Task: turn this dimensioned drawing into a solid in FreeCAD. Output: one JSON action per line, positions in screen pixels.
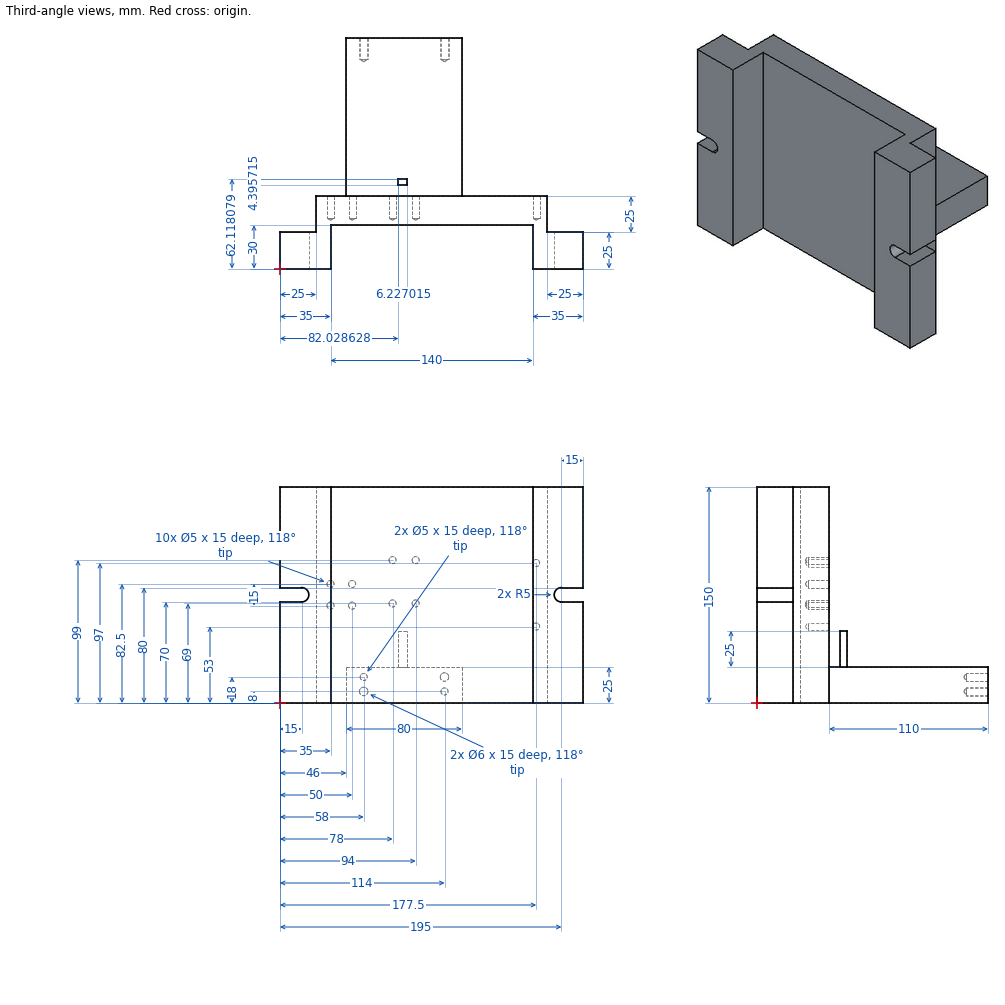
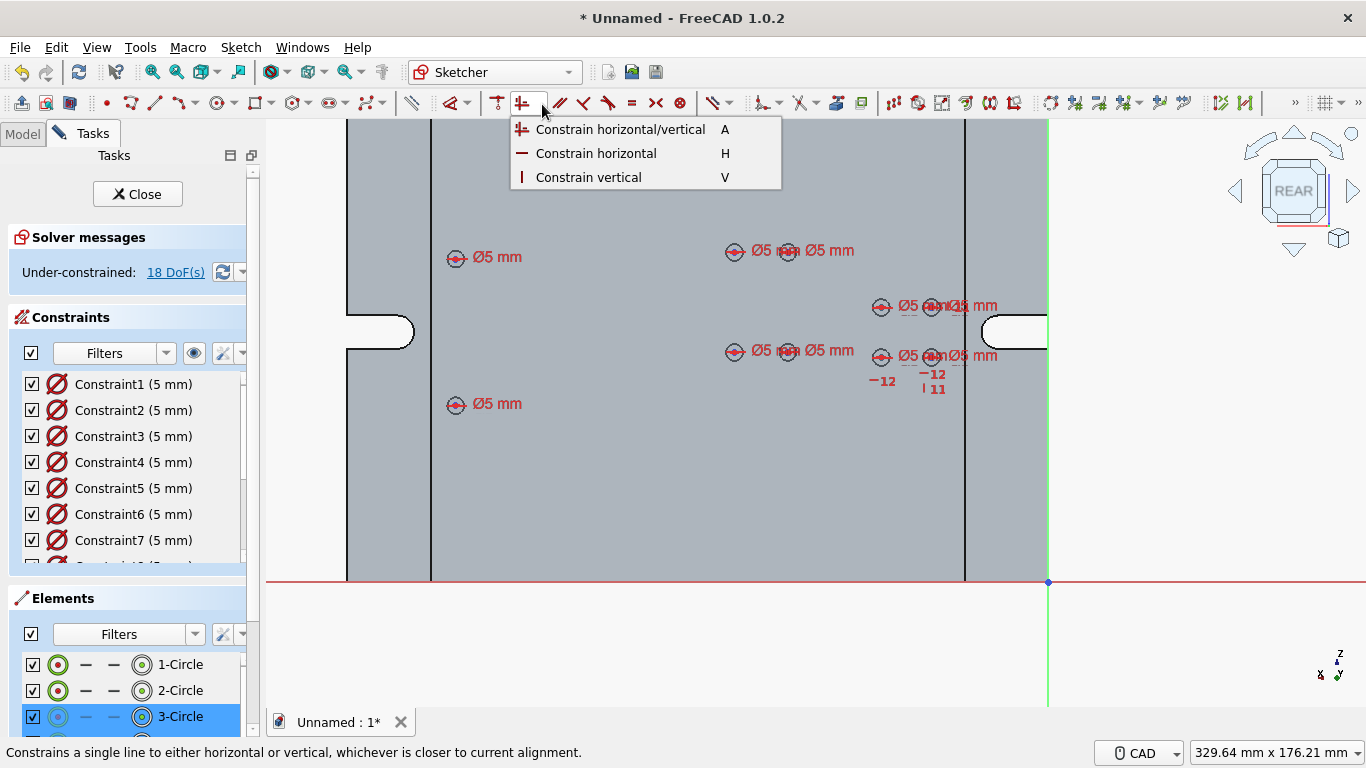
{"action": "left_click", "coordinate": [646, 177]}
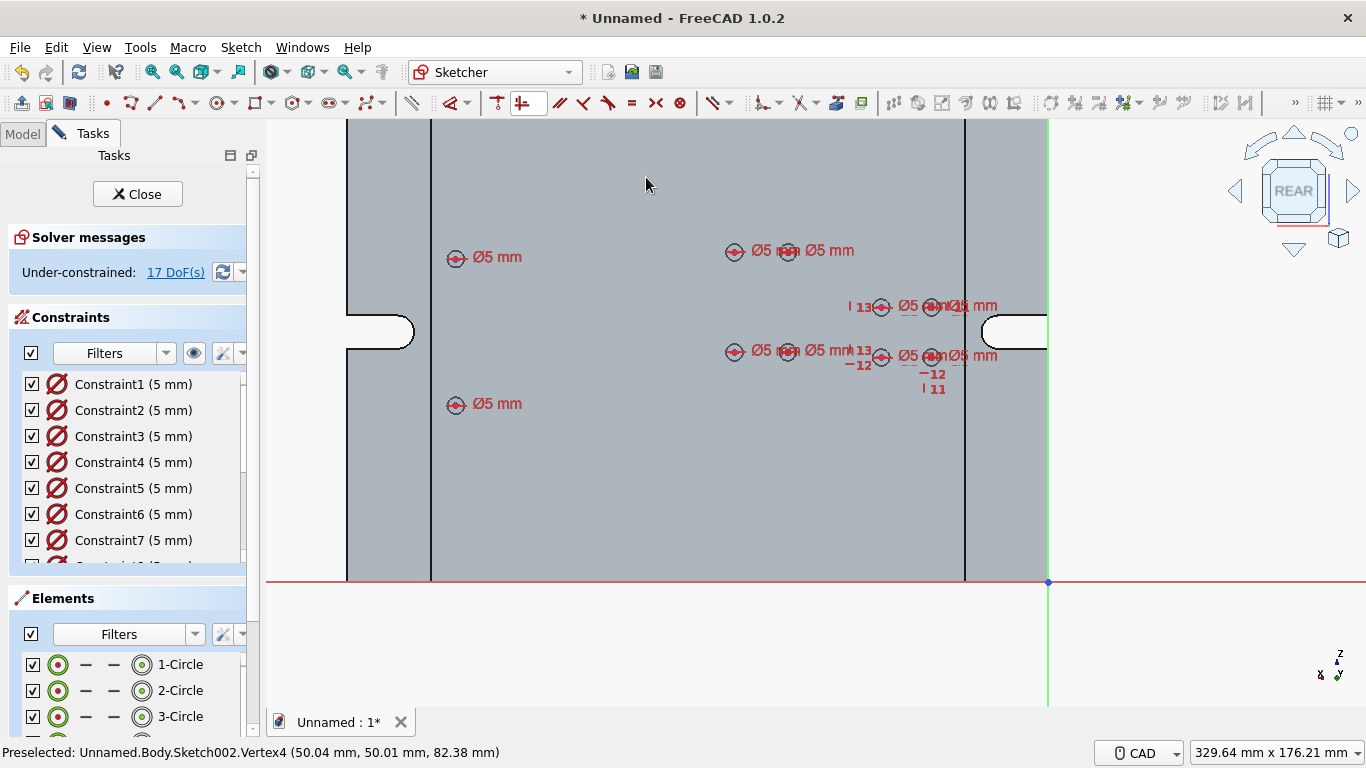
{"action": "left_click", "coordinate": [932, 308]}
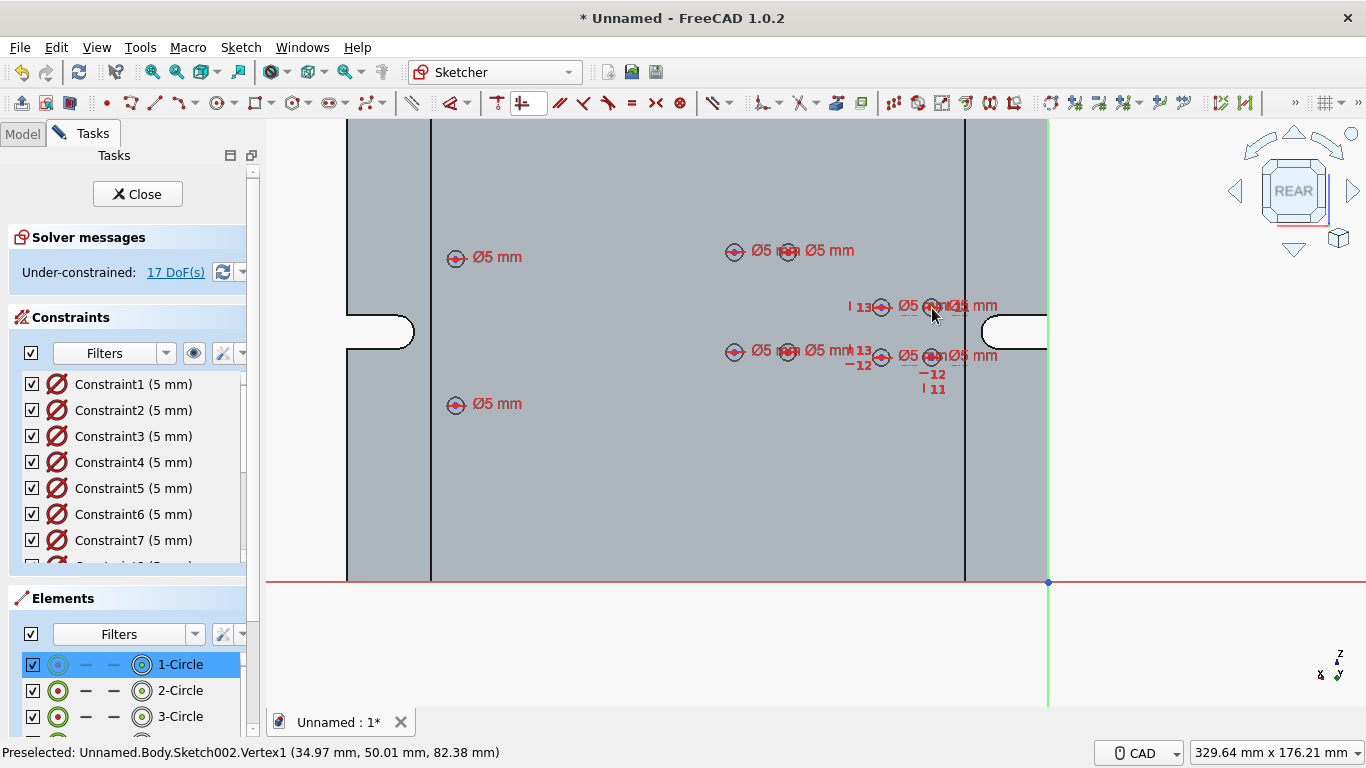
{"action": "left_click", "coordinate": [881, 308]}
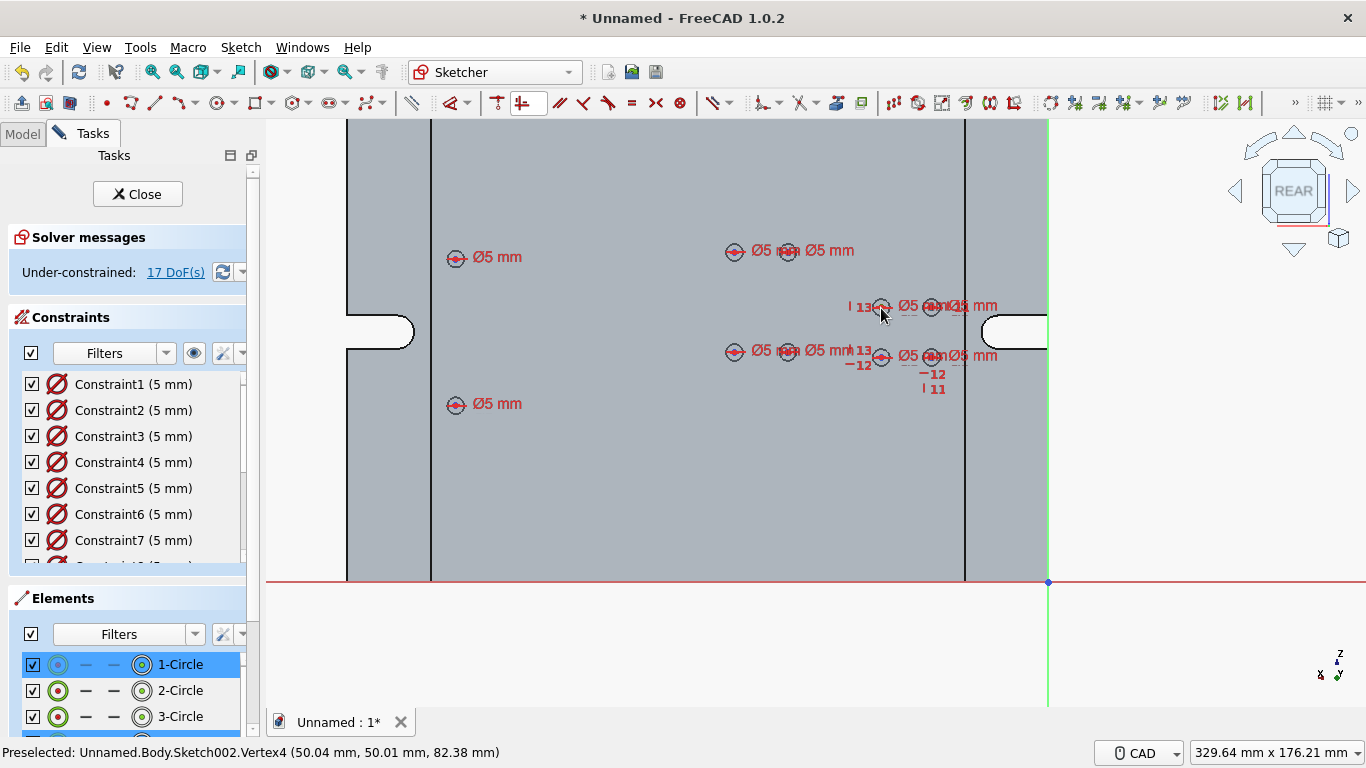
{"action": "left_click", "coordinate": [542, 104]}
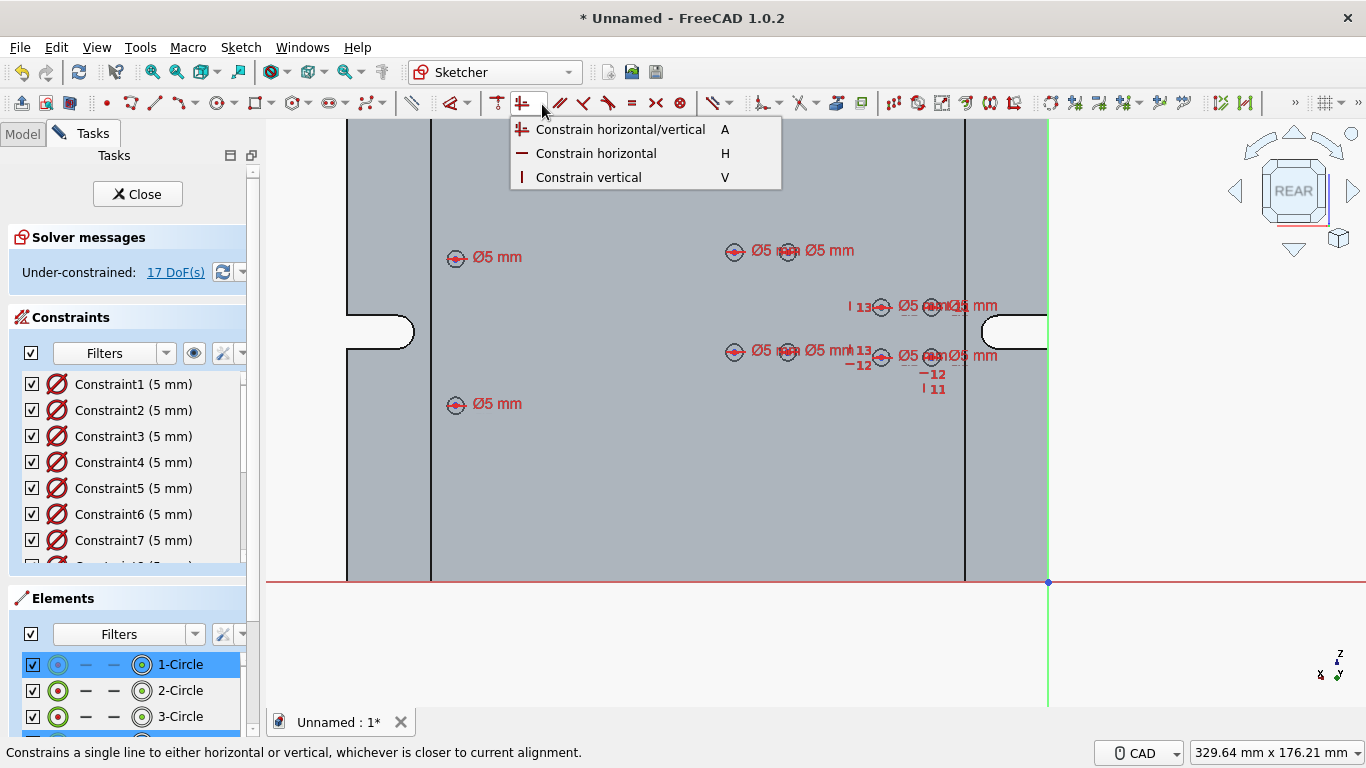
{"action": "left_click", "coordinate": [646, 153]}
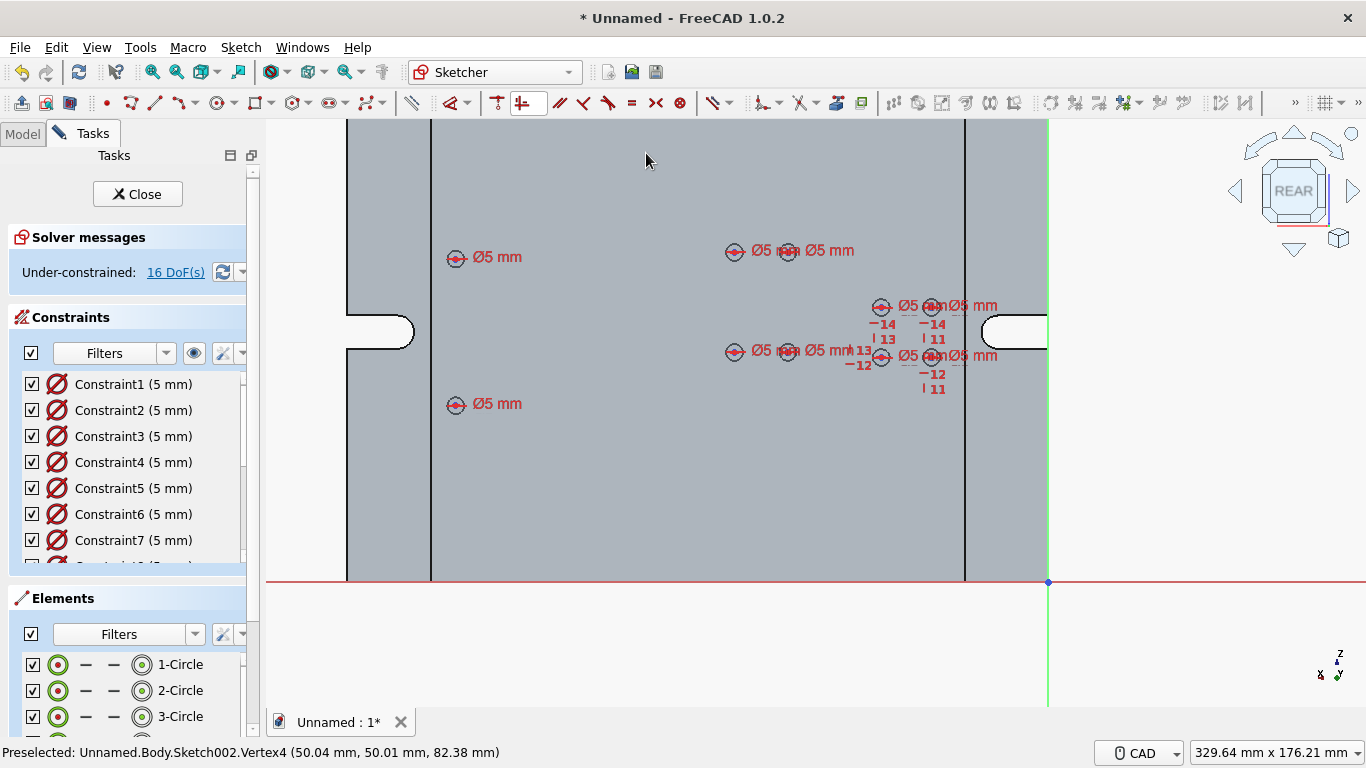
{"action": "left_click", "coordinate": [788, 352]}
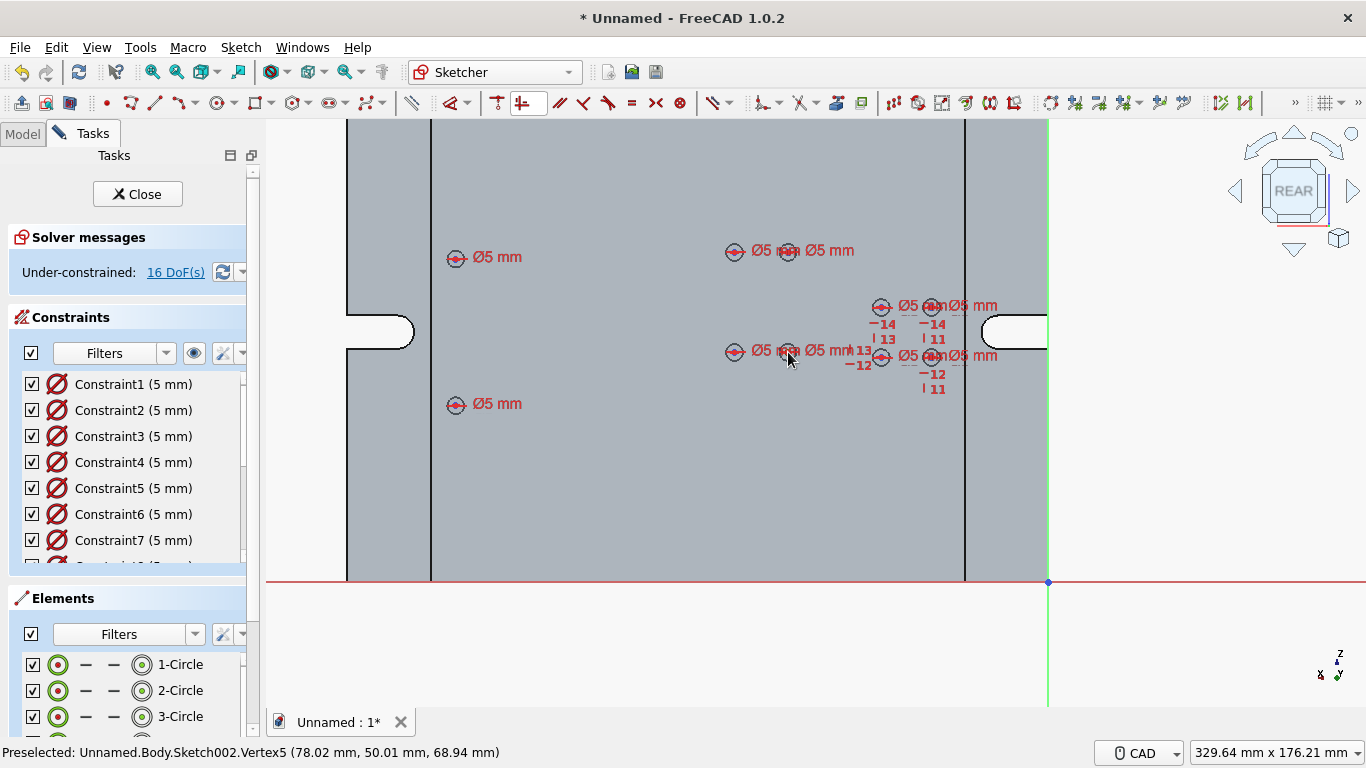
{"action": "left_click", "coordinate": [788, 252]}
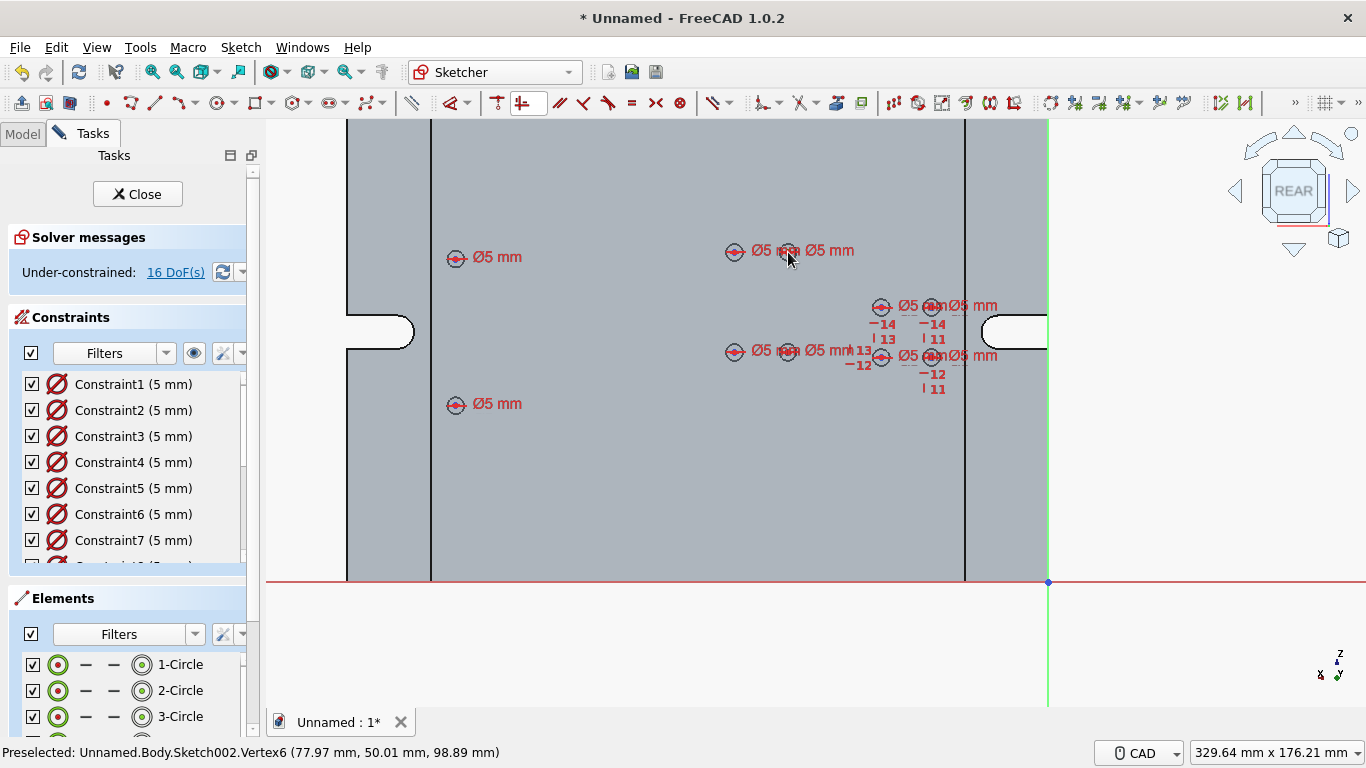
{"action": "left_click", "coordinate": [542, 104]}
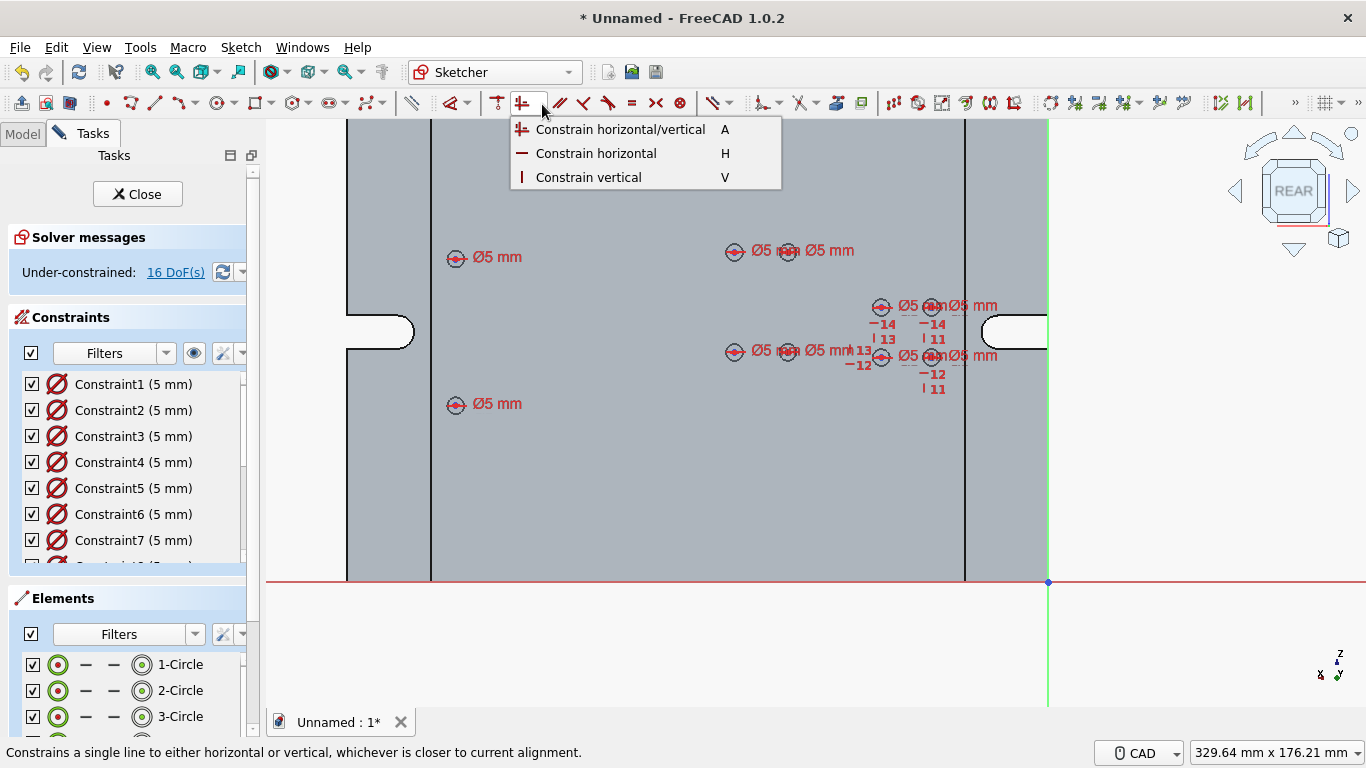
{"action": "left_click", "coordinate": [646, 177]}